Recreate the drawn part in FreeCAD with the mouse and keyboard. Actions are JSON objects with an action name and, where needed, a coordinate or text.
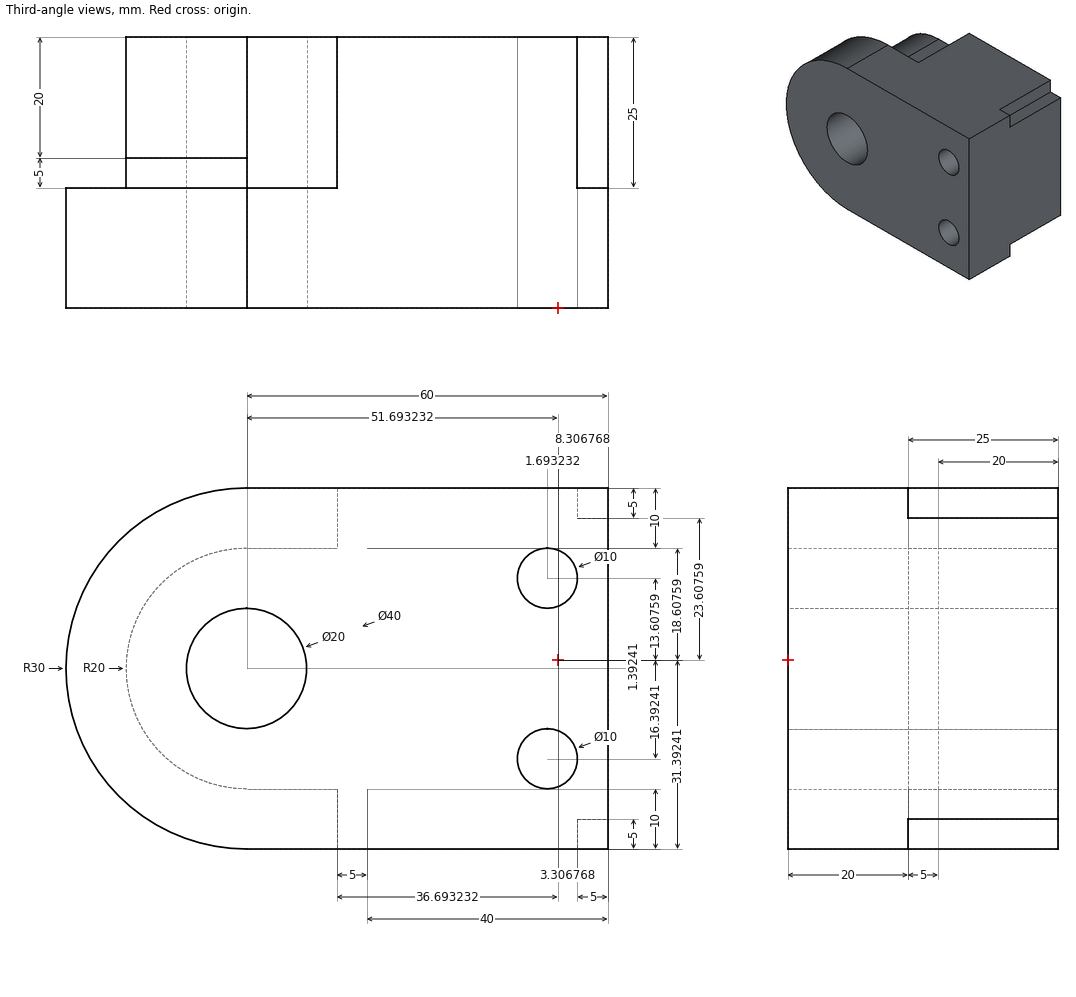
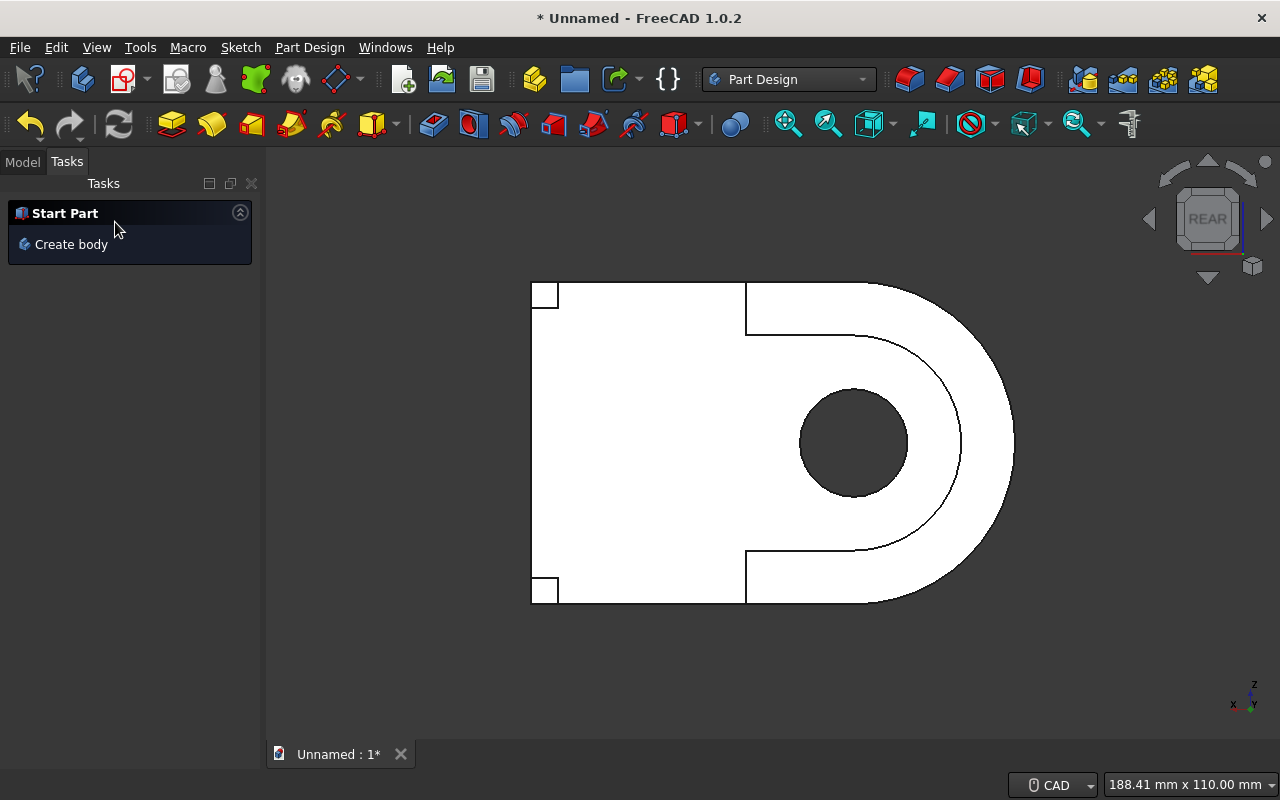
{"action": "left_click", "coordinate": [685, 442]}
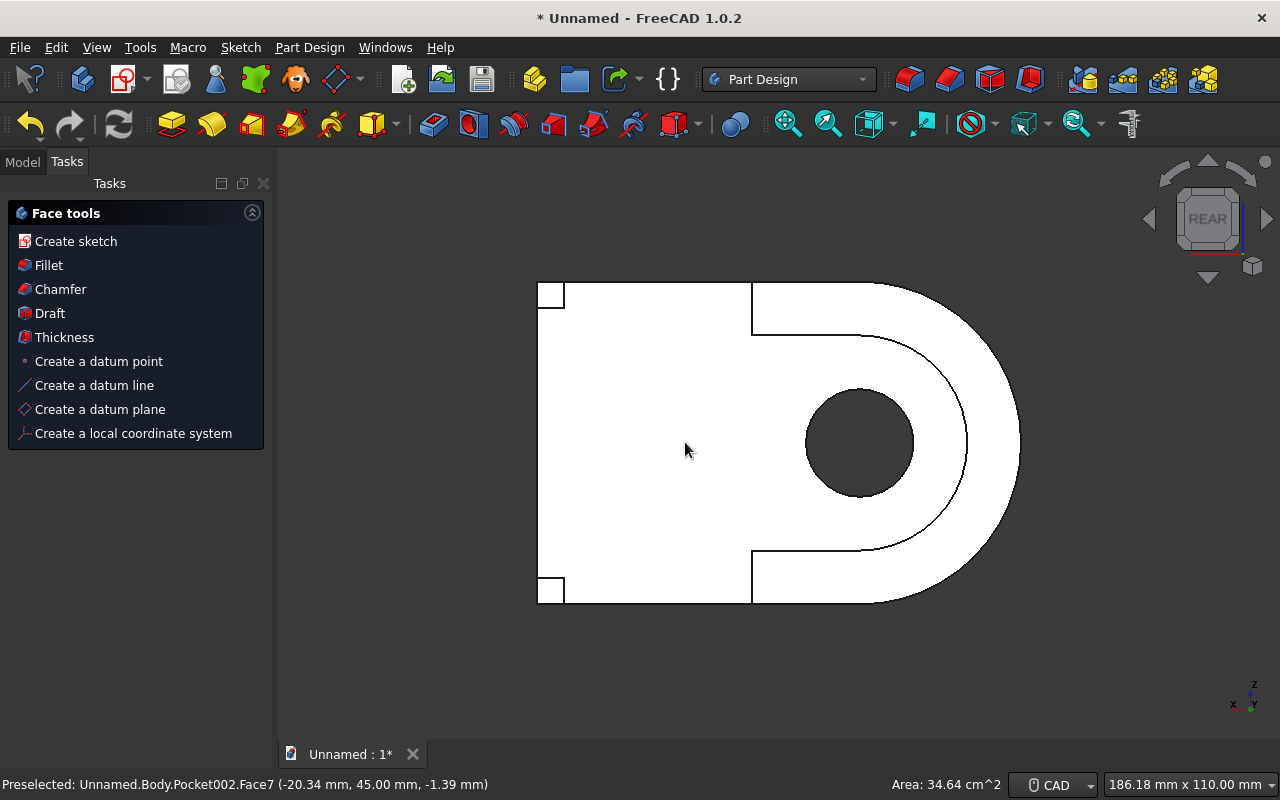
{"action": "left_click", "coordinate": [124, 80]}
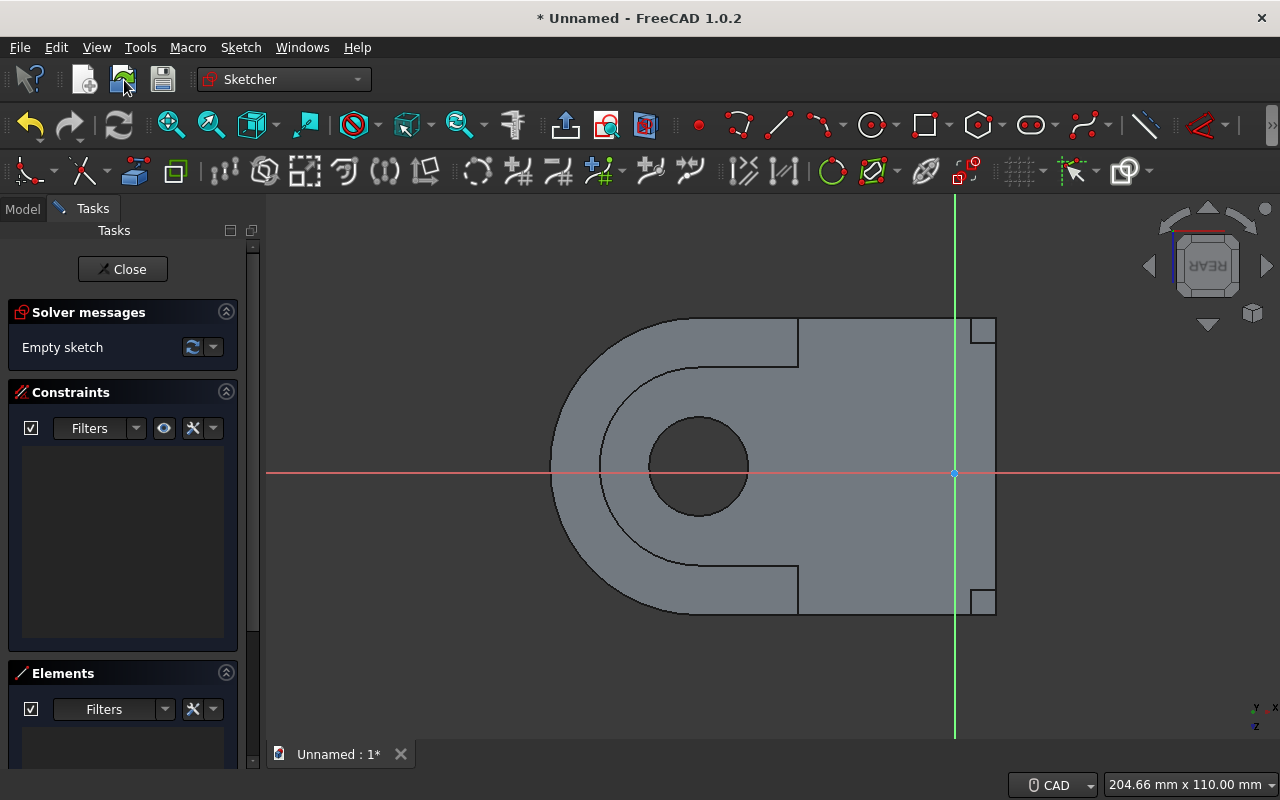
{"action": "scroll", "coordinate": [1026, 537], "scroll_direction": "up", "scroll_amount": 7}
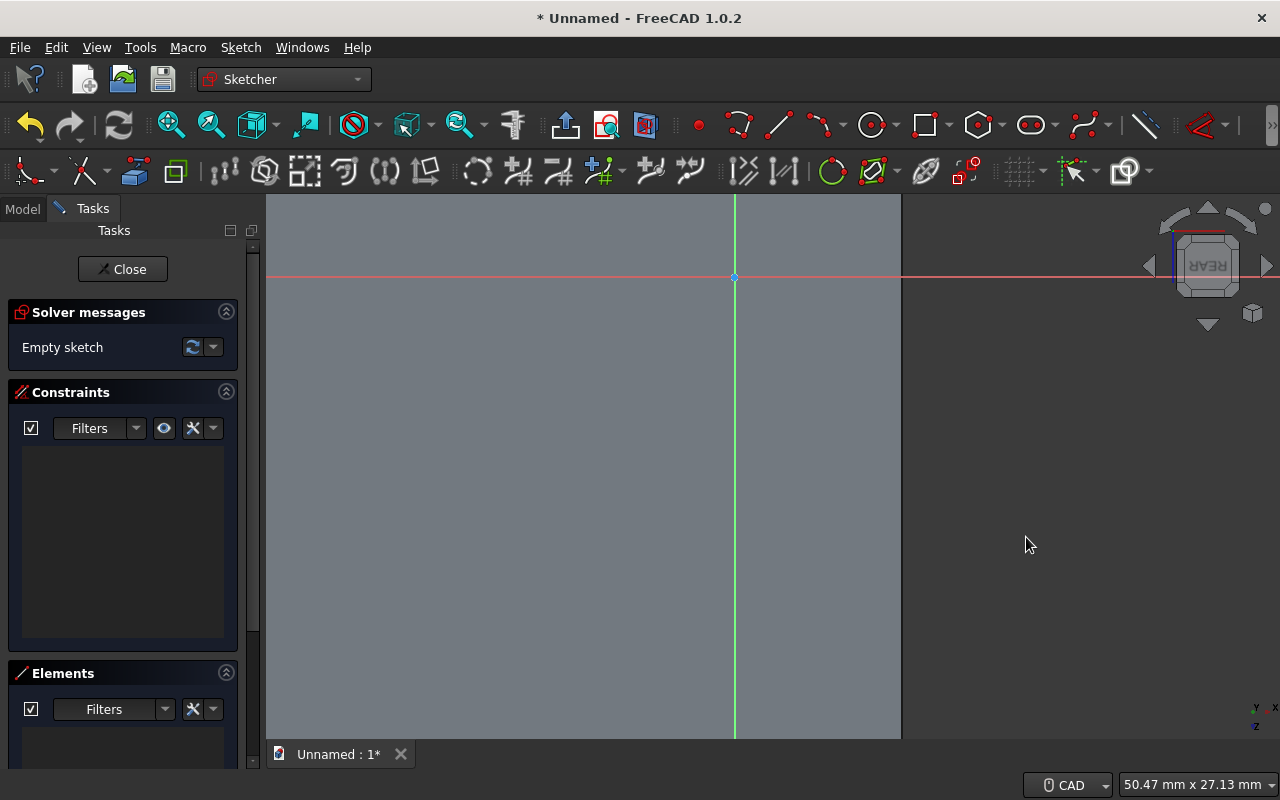
{"action": "left_click", "coordinate": [872, 126]}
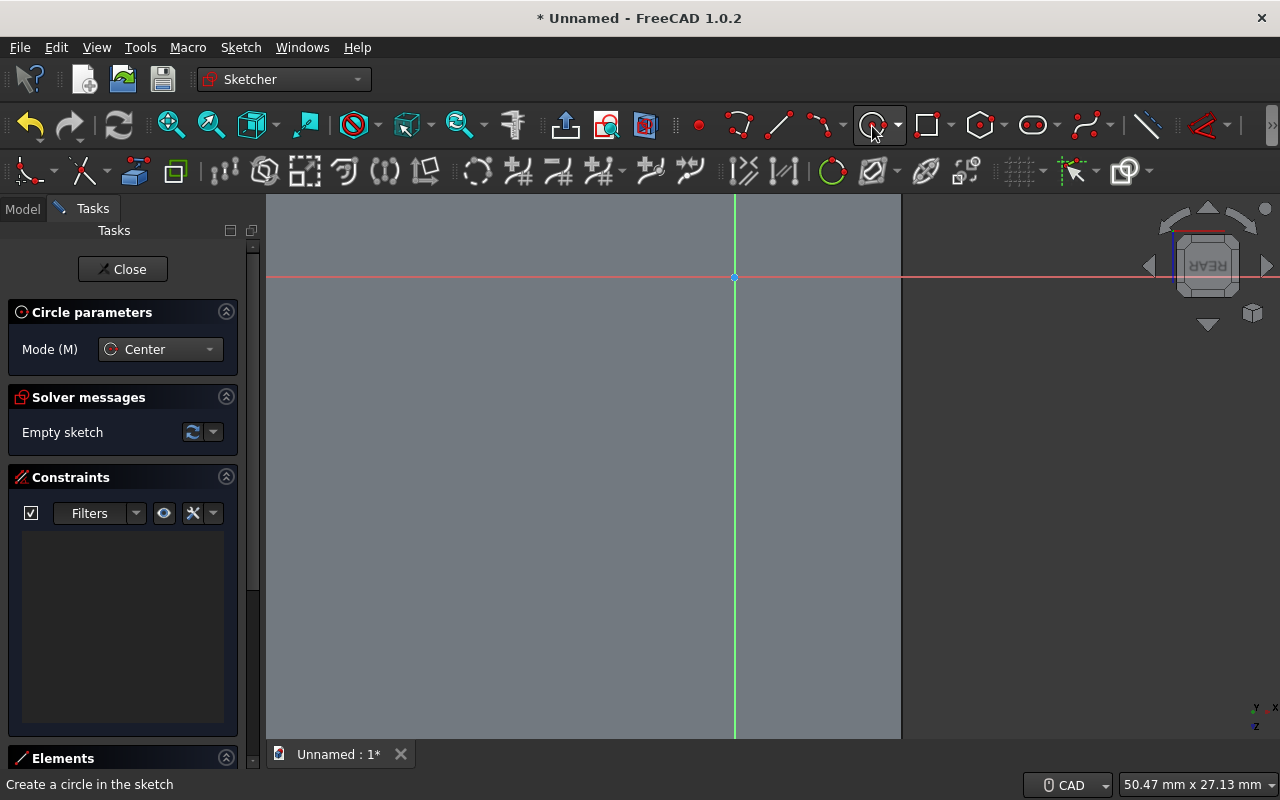
{"action": "left_click", "coordinate": [701, 551]}
{"action": "left_click", "coordinate": [772, 480]}
{"action": "key", "text": "Escape"}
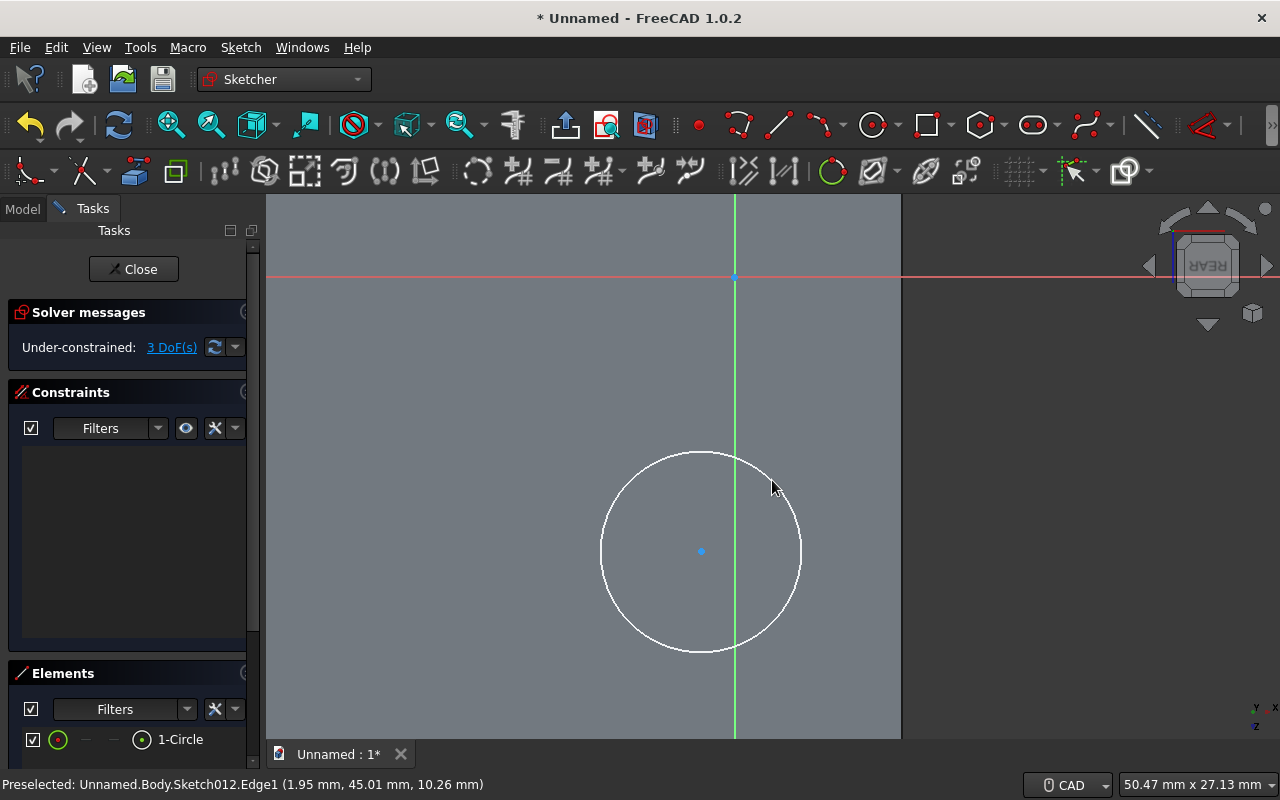
{"action": "key", "text": "d"}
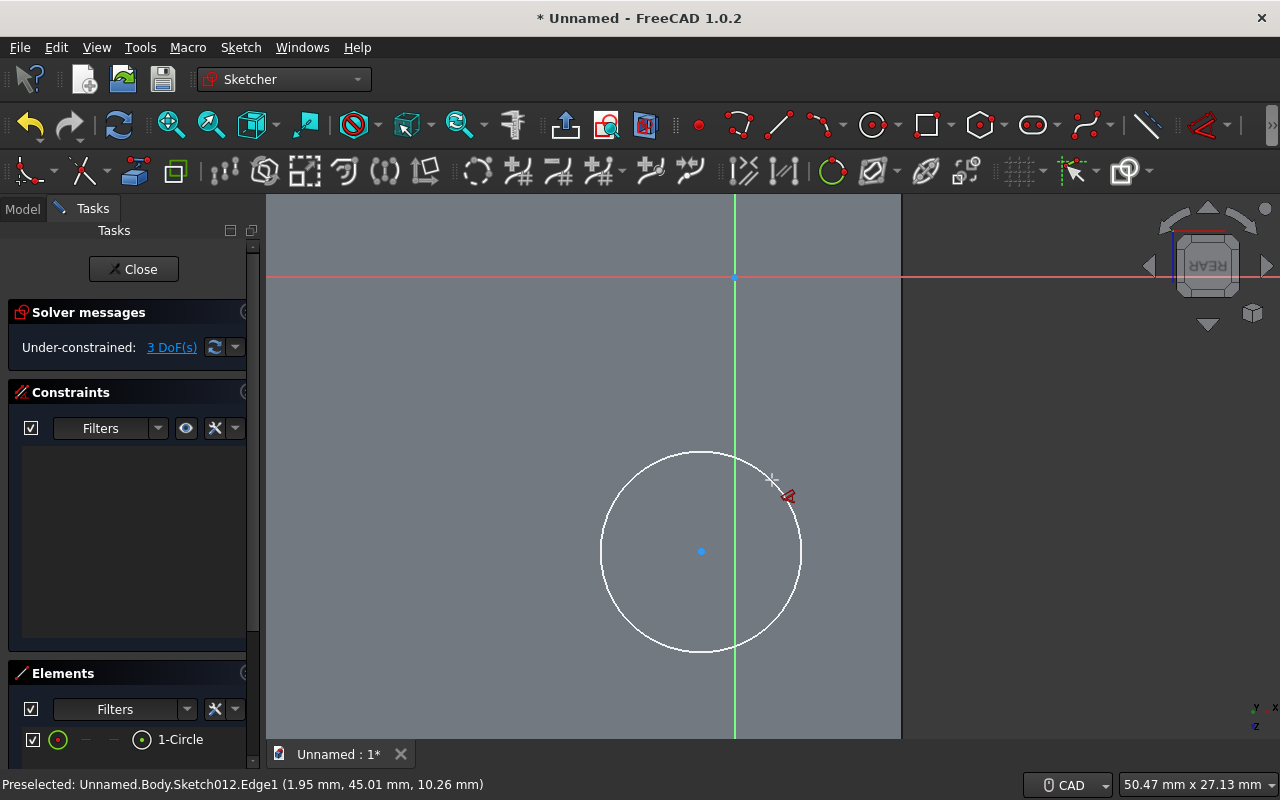
{"action": "left_click", "coordinate": [772, 481]}
{"action": "left_click", "coordinate": [795, 458]}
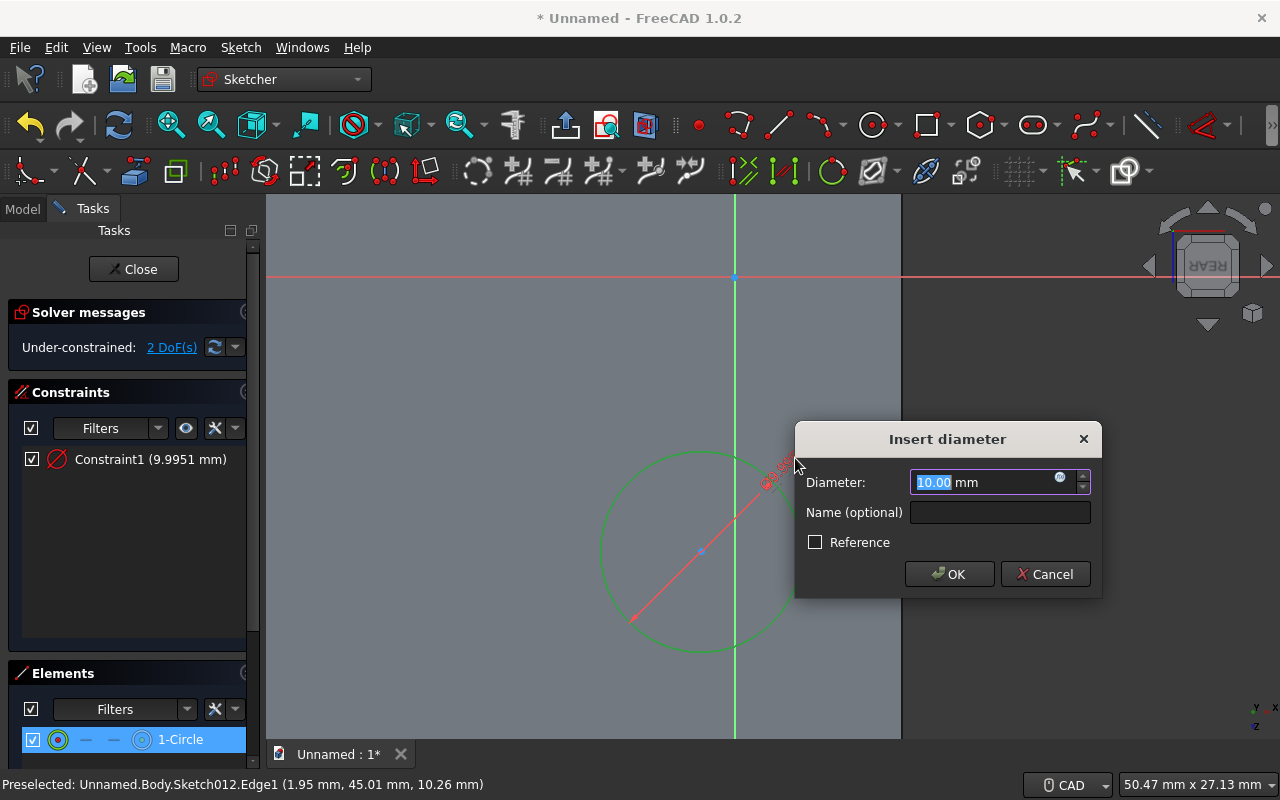
{"action": "type", "text": "10"}
{"action": "key", "text": "Return"}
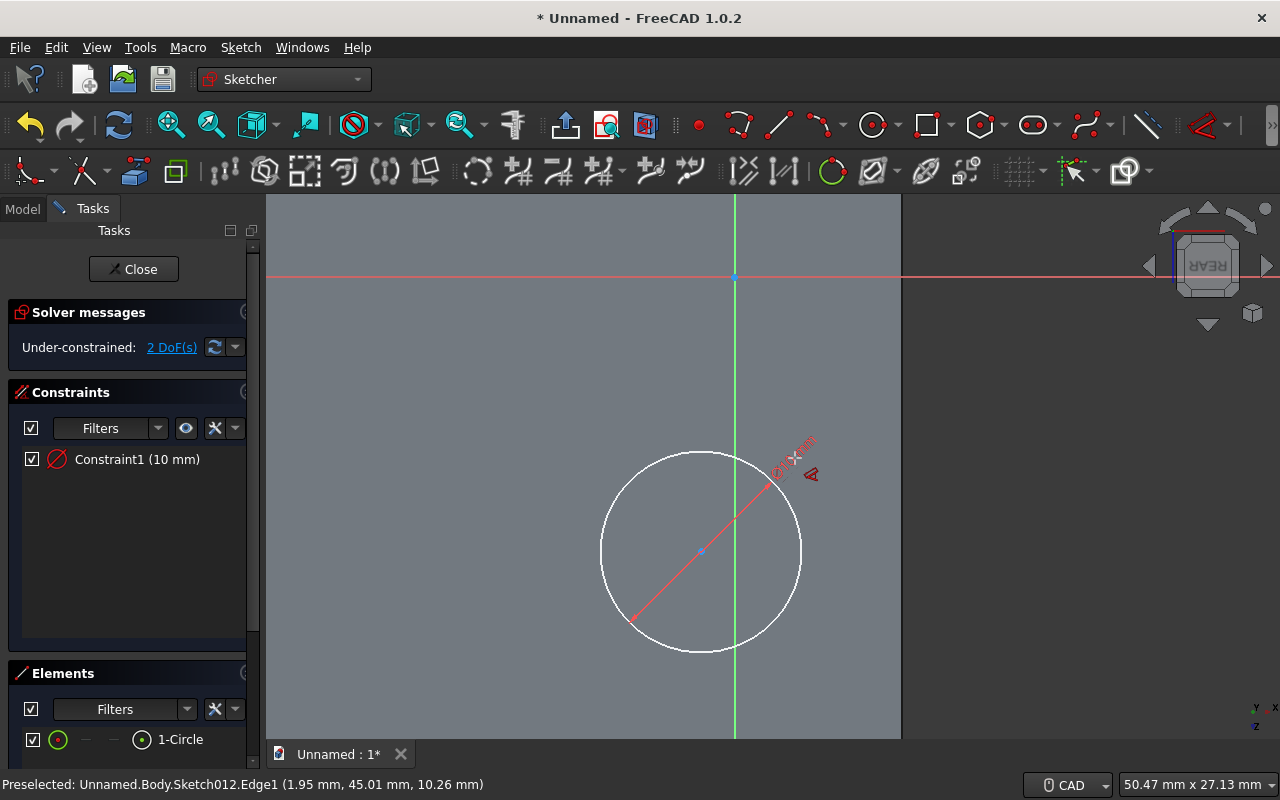
{"action": "left_click", "coordinate": [701, 552]}
{"action": "left_click", "coordinate": [718, 243]}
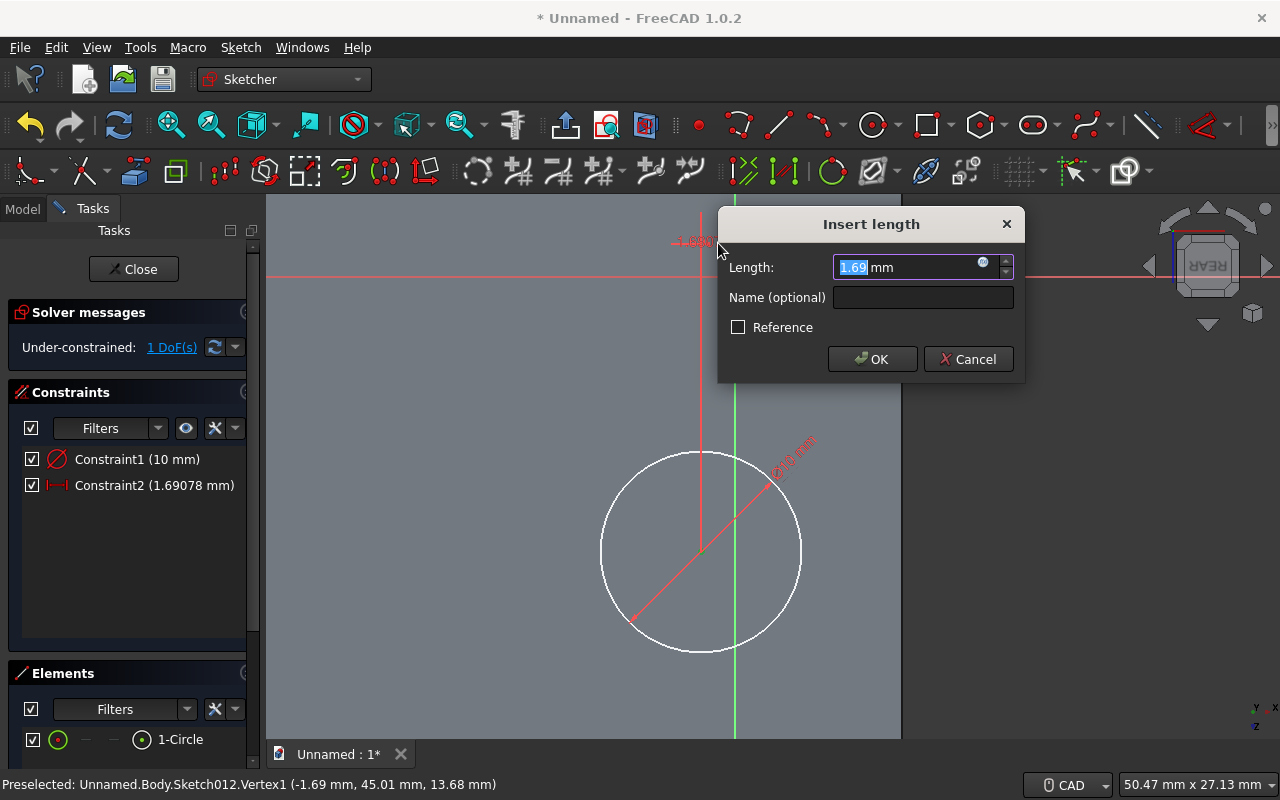
{"action": "type", "text": "1.693232"}
{"action": "key", "text": "Return"}